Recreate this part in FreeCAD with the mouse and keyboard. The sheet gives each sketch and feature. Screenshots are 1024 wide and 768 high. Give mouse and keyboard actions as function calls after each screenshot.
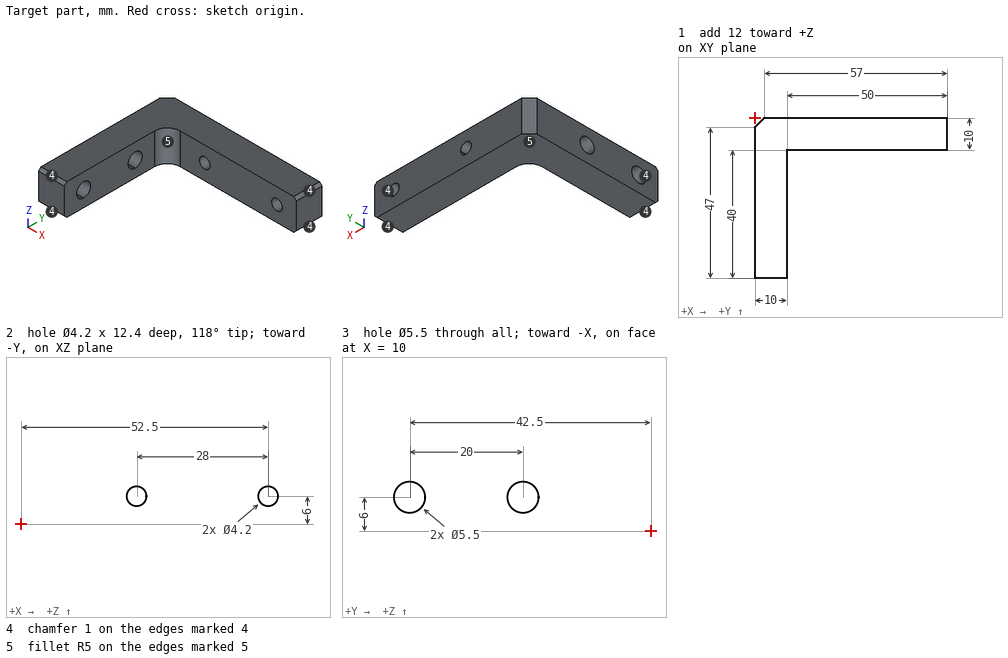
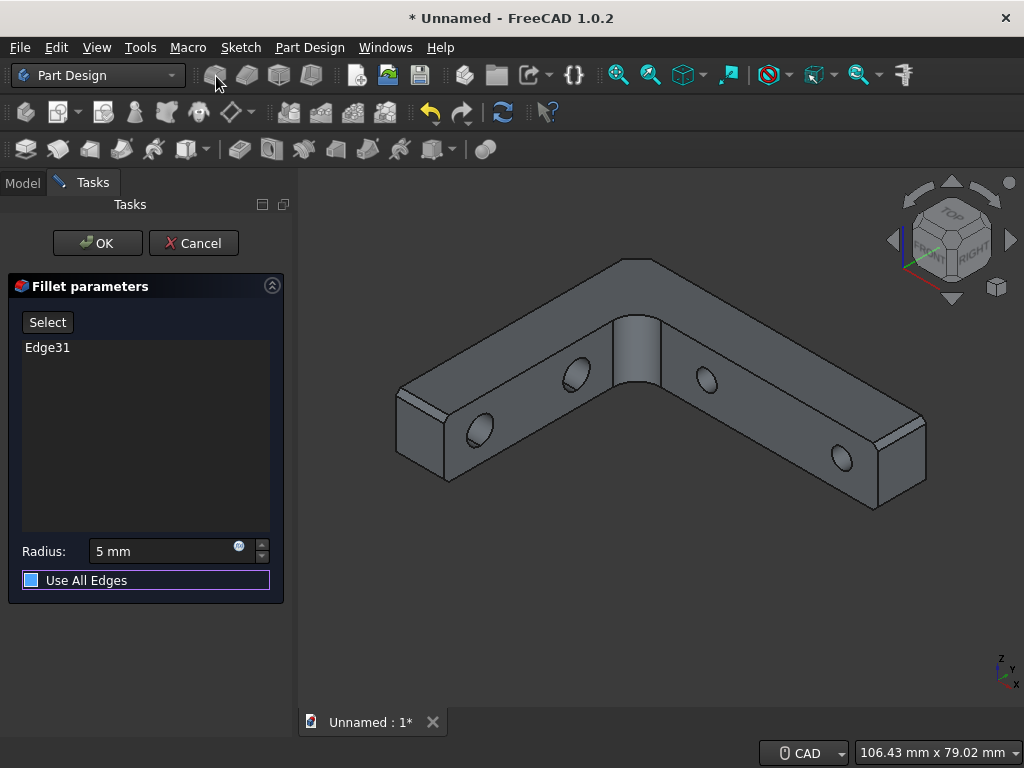
click(98, 243)